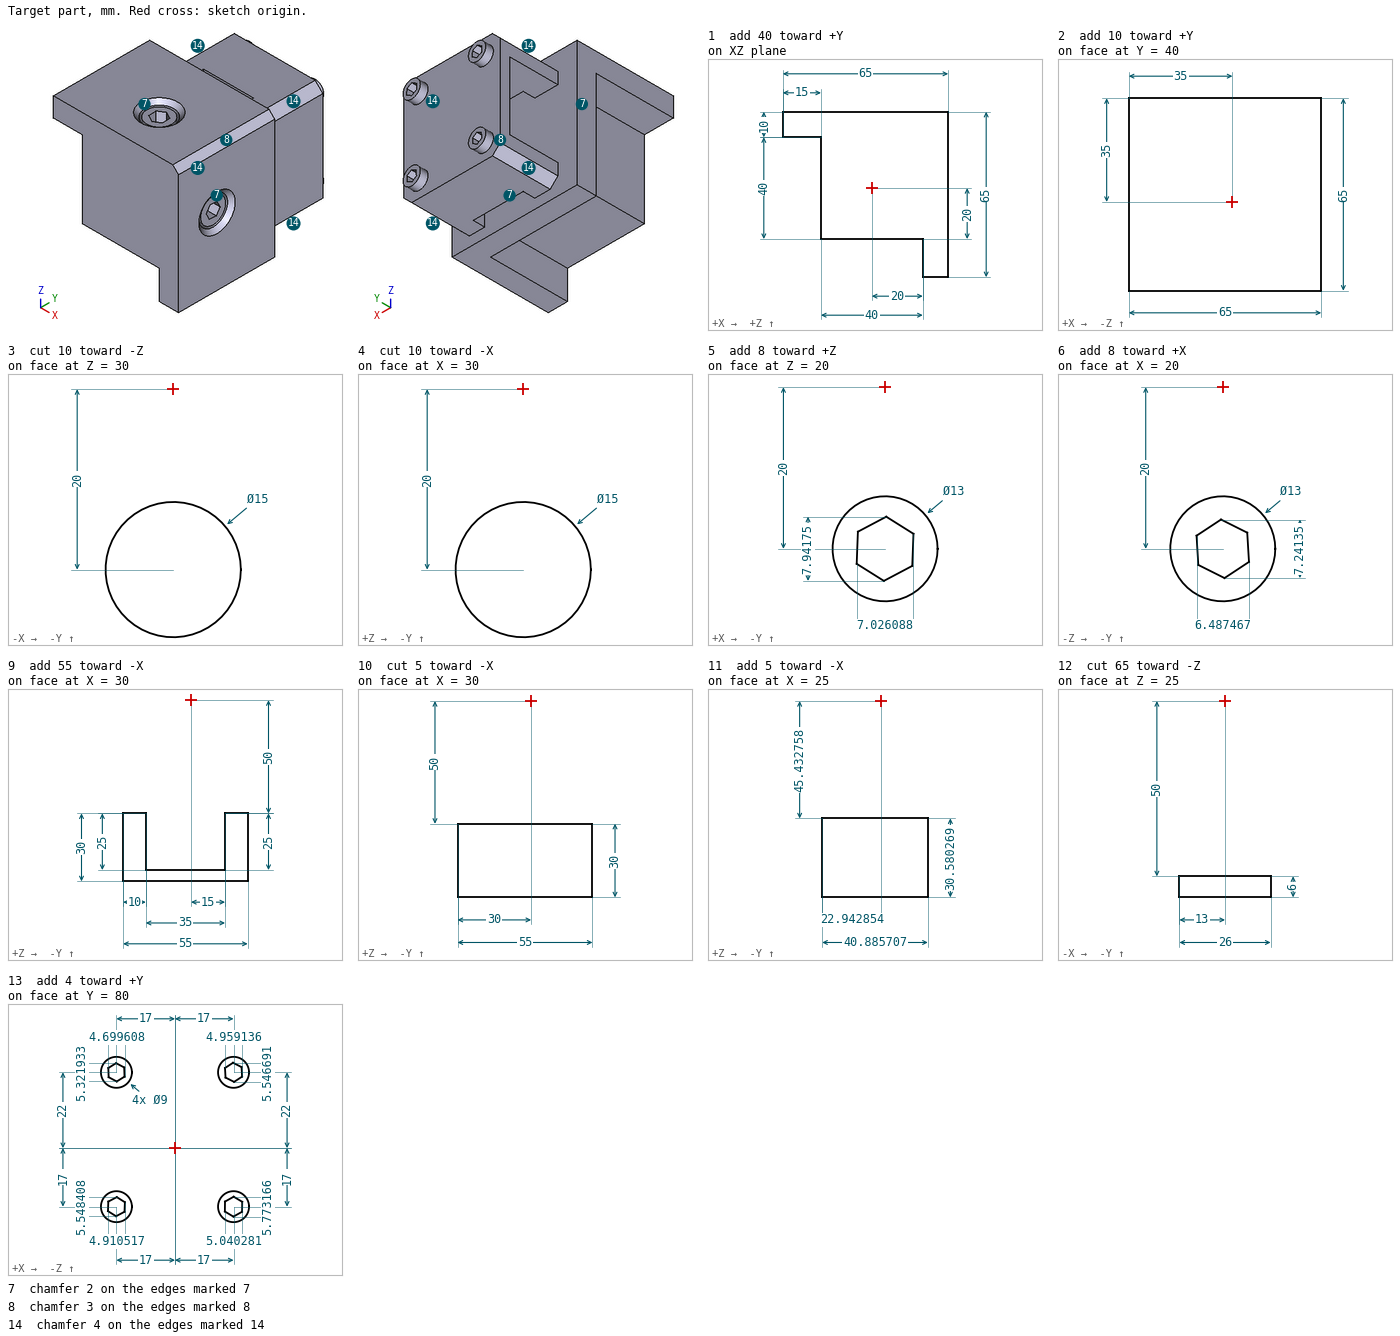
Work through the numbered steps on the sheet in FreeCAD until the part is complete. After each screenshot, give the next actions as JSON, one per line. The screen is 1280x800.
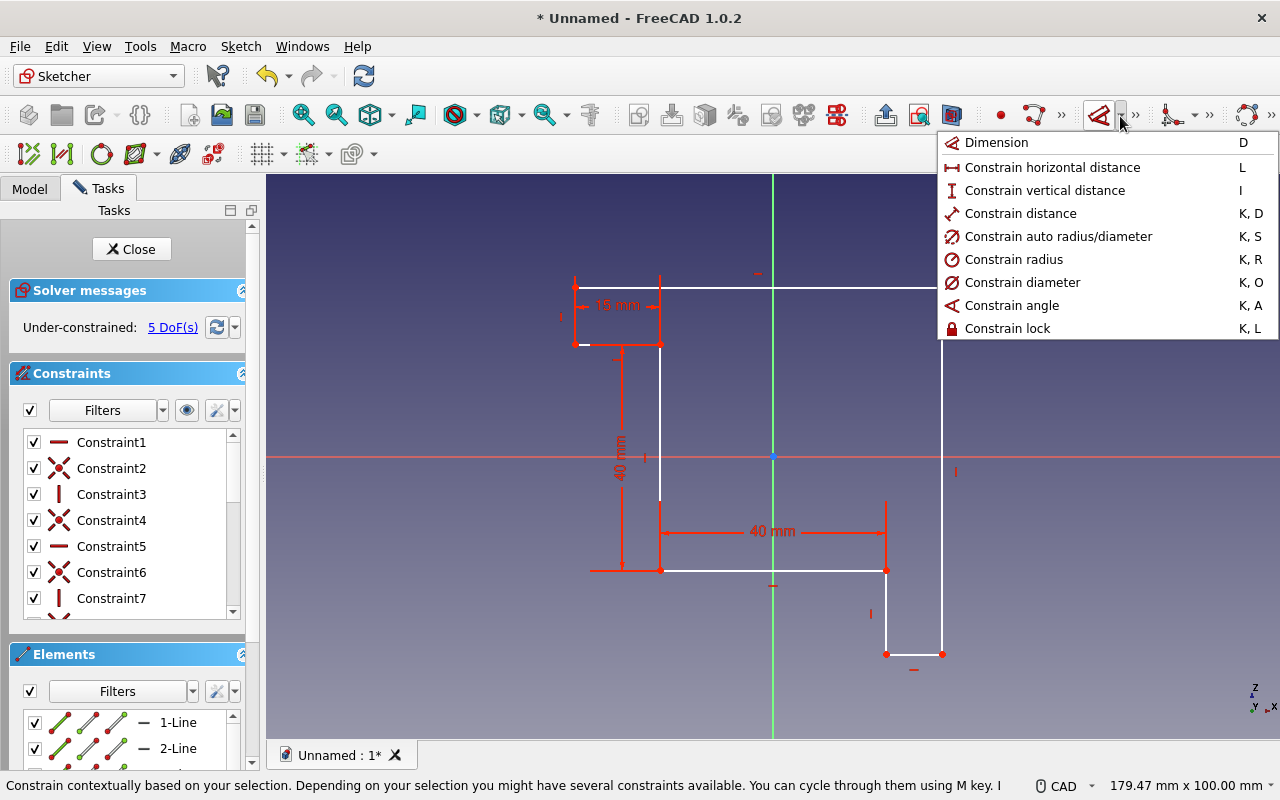
{"action": "left_click", "coordinate": [1108, 190]}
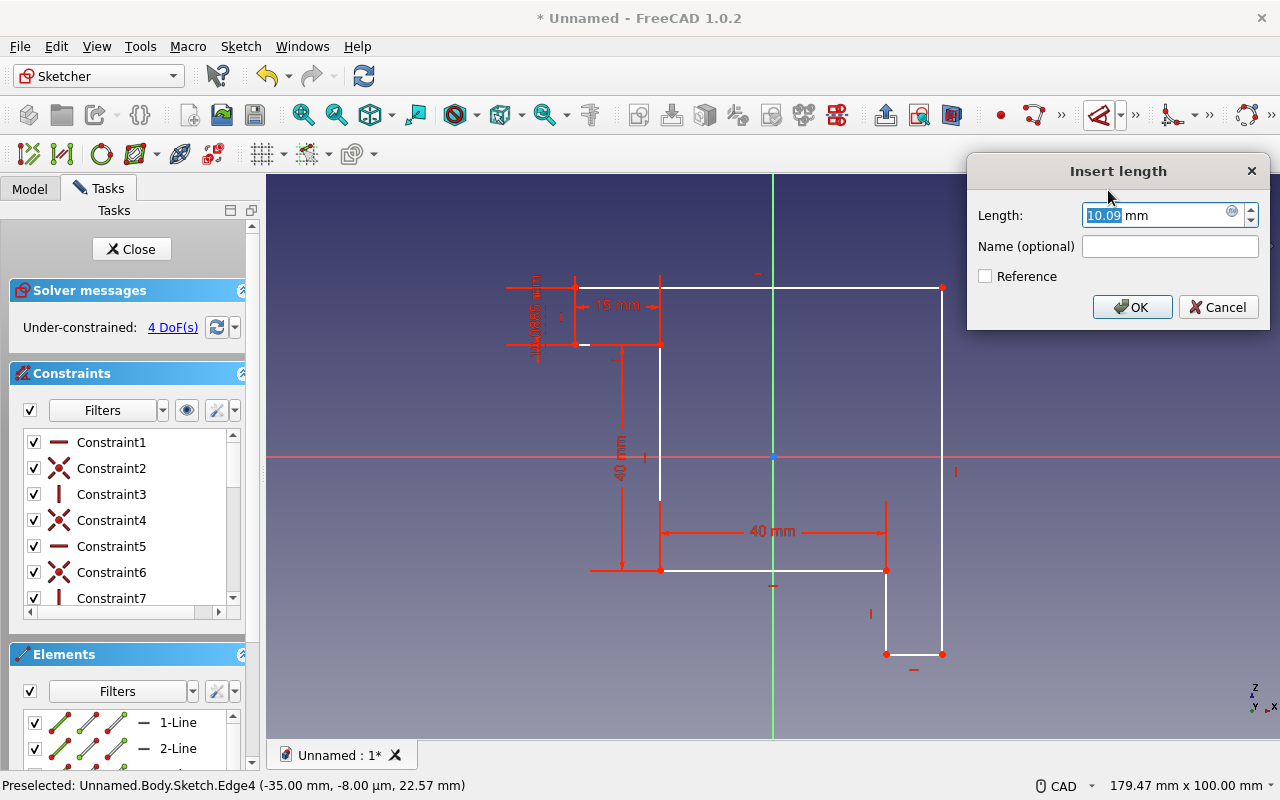
{"action": "type", "text": "10"}
{"action": "key", "text": "Return"}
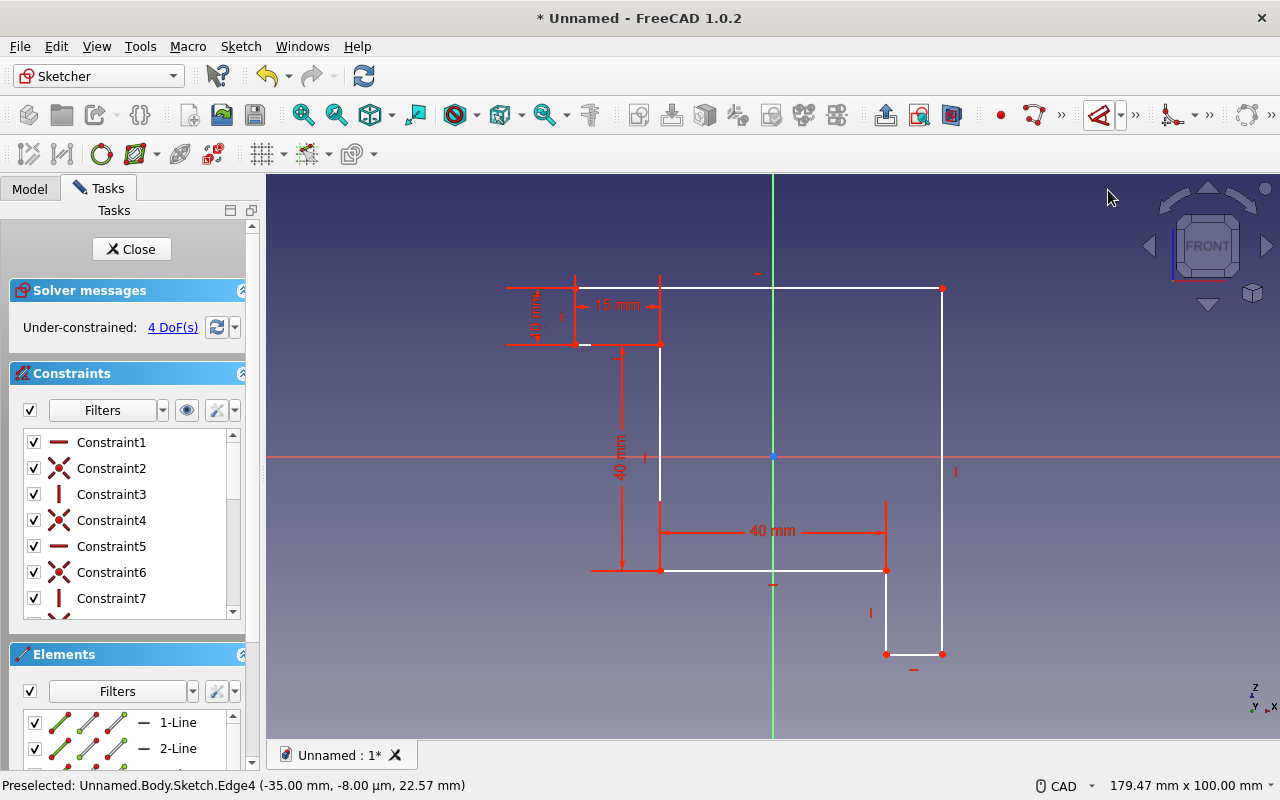
{"action": "left_click", "coordinate": [685, 288]}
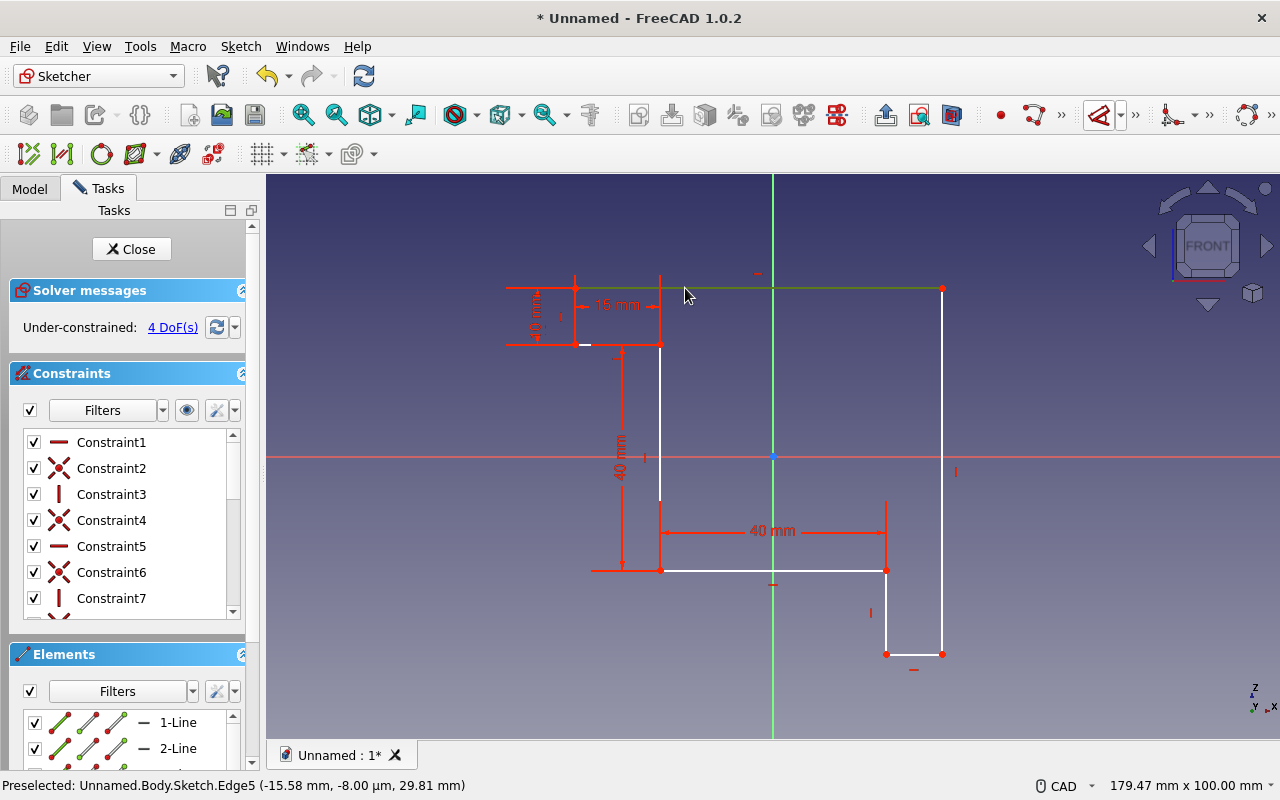
{"action": "key", "text": "l"}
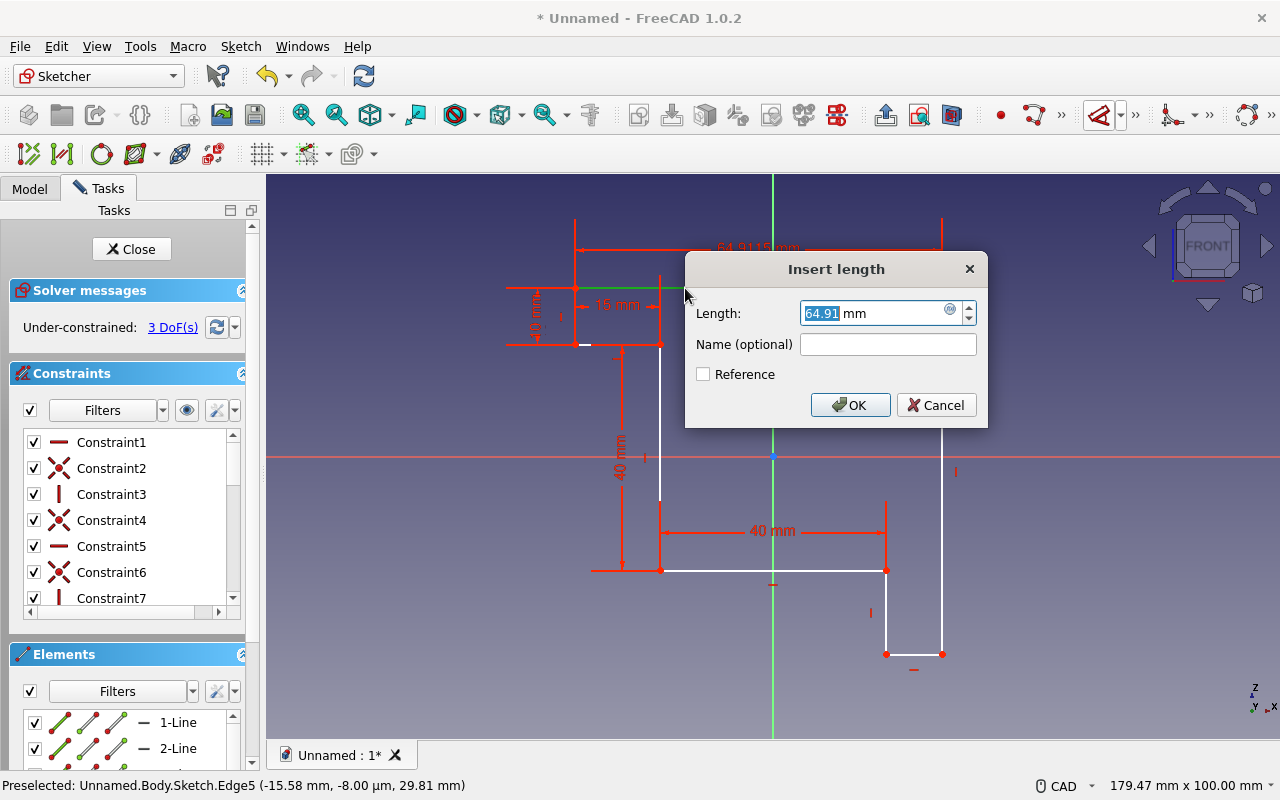
{"action": "type", "text": "65"}
{"action": "key", "text": "Return"}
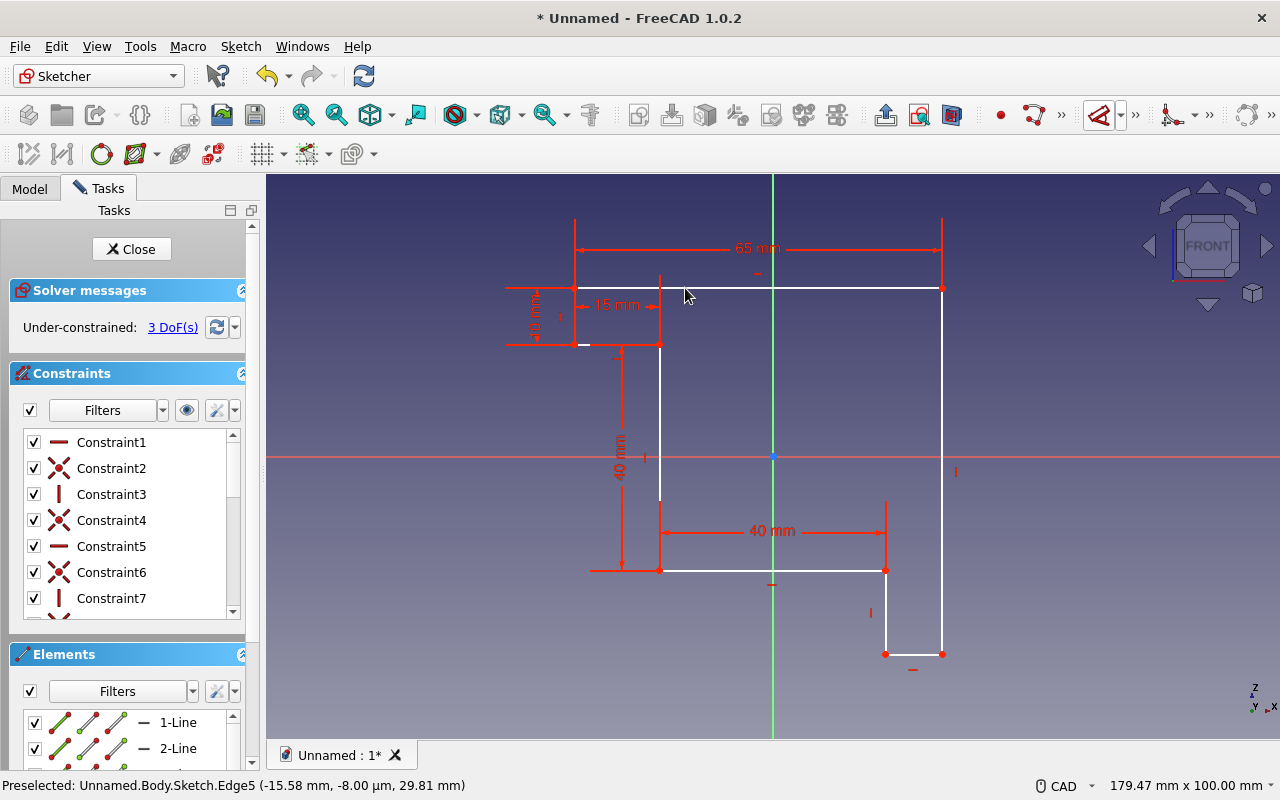
{"action": "left_click", "coordinate": [942, 398]}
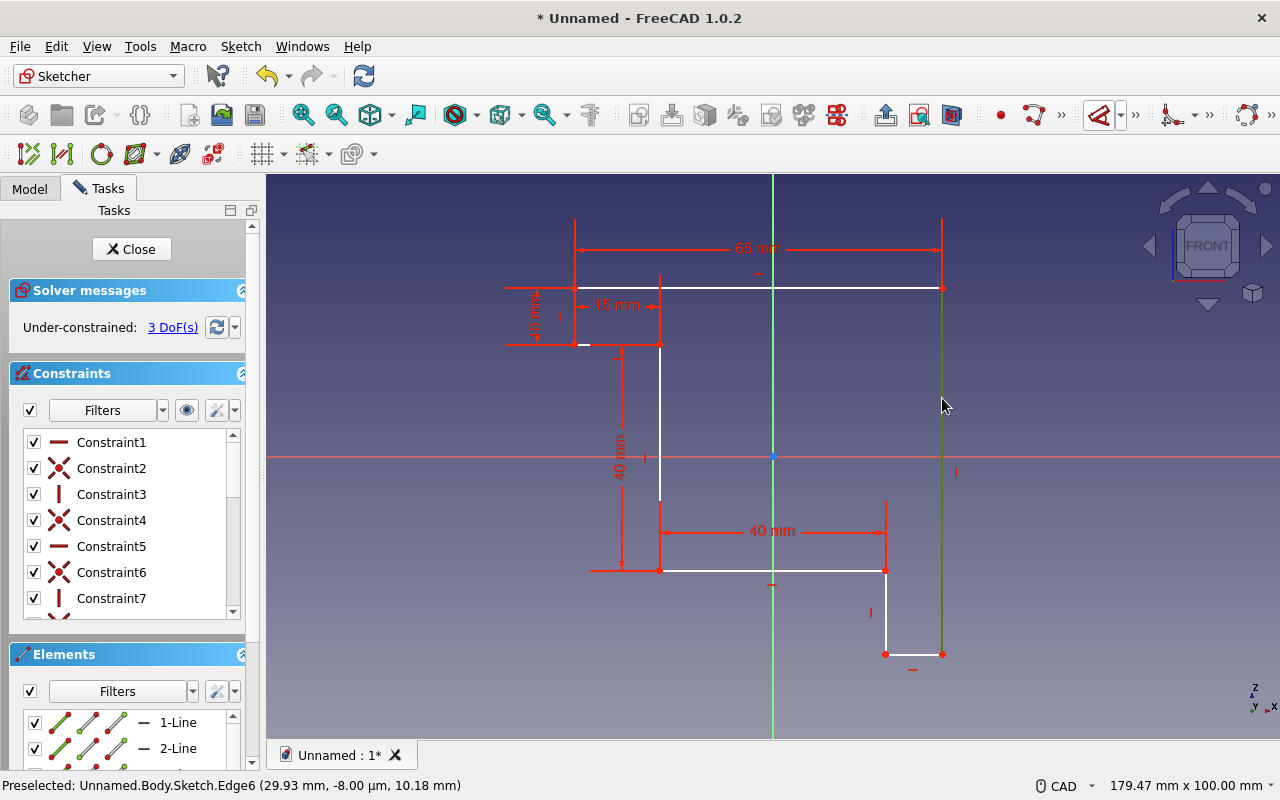
{"action": "left_click", "coordinate": [1120, 116]}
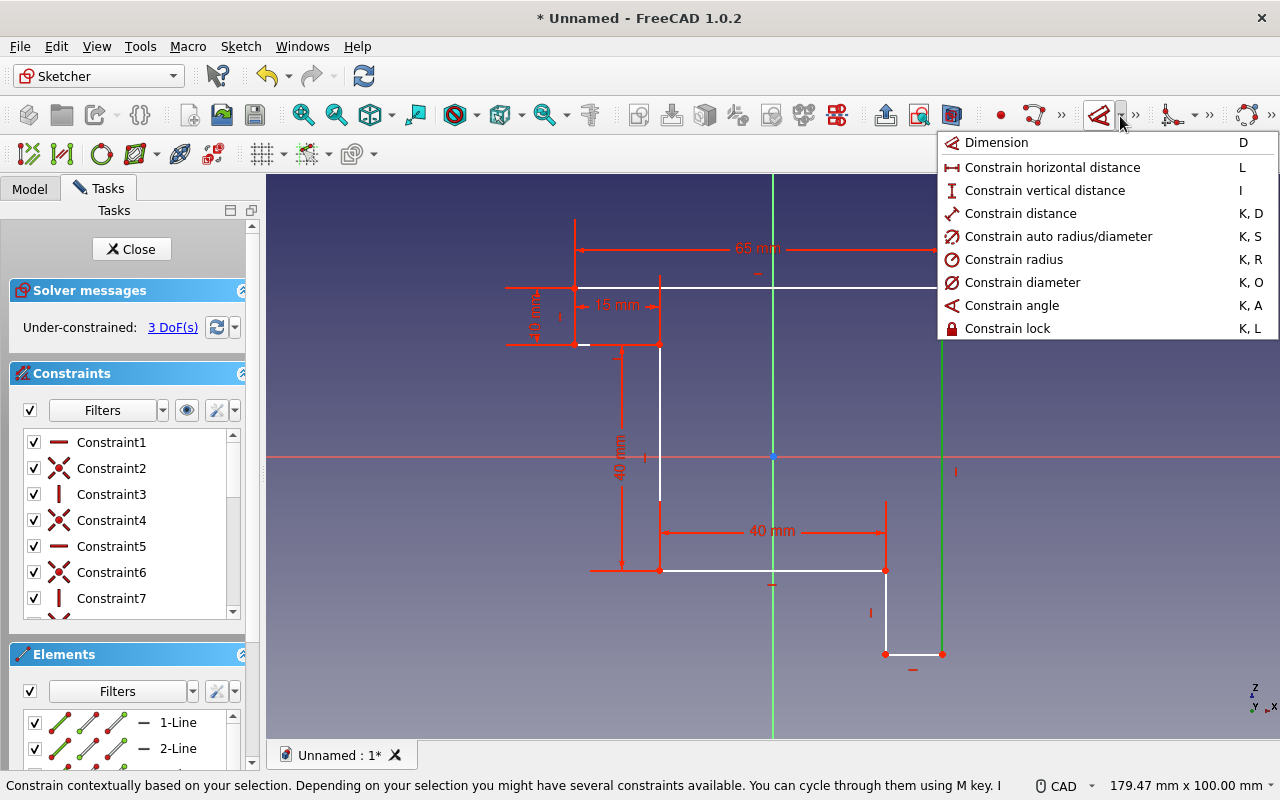
{"action": "left_click", "coordinate": [1108, 190]}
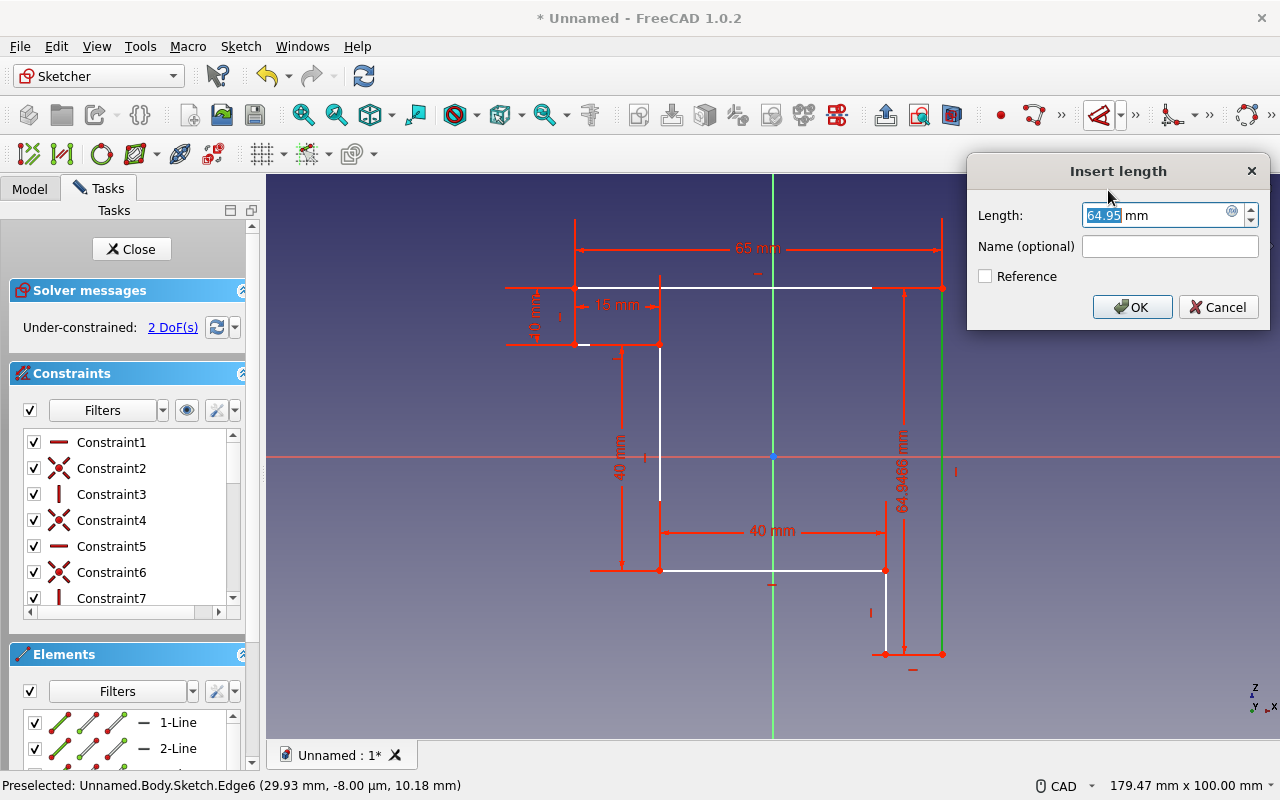
{"action": "type", "text": "65"}
{"action": "key", "text": "Return"}